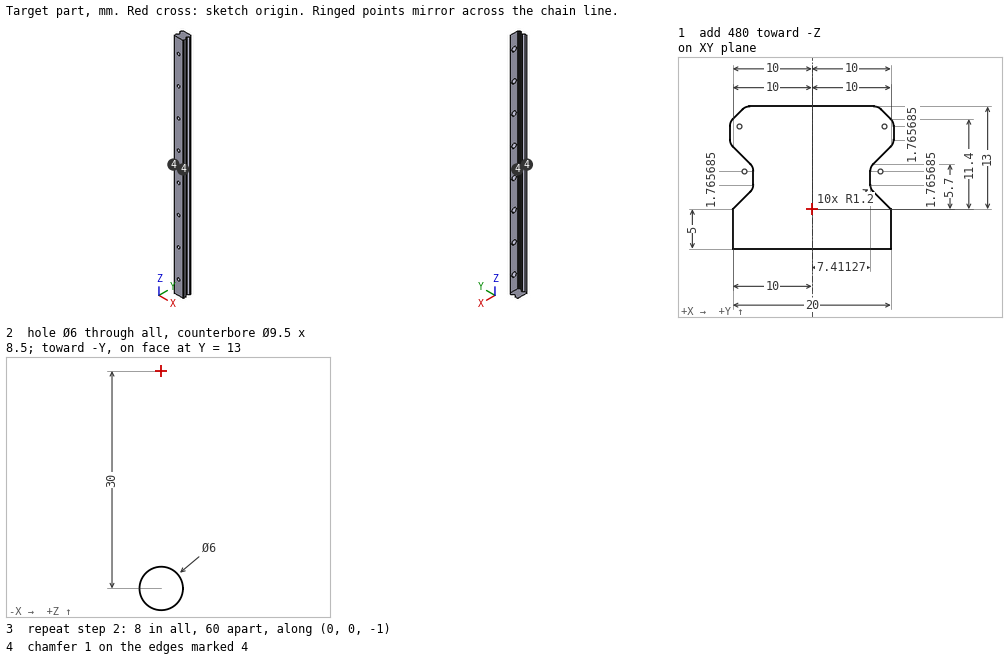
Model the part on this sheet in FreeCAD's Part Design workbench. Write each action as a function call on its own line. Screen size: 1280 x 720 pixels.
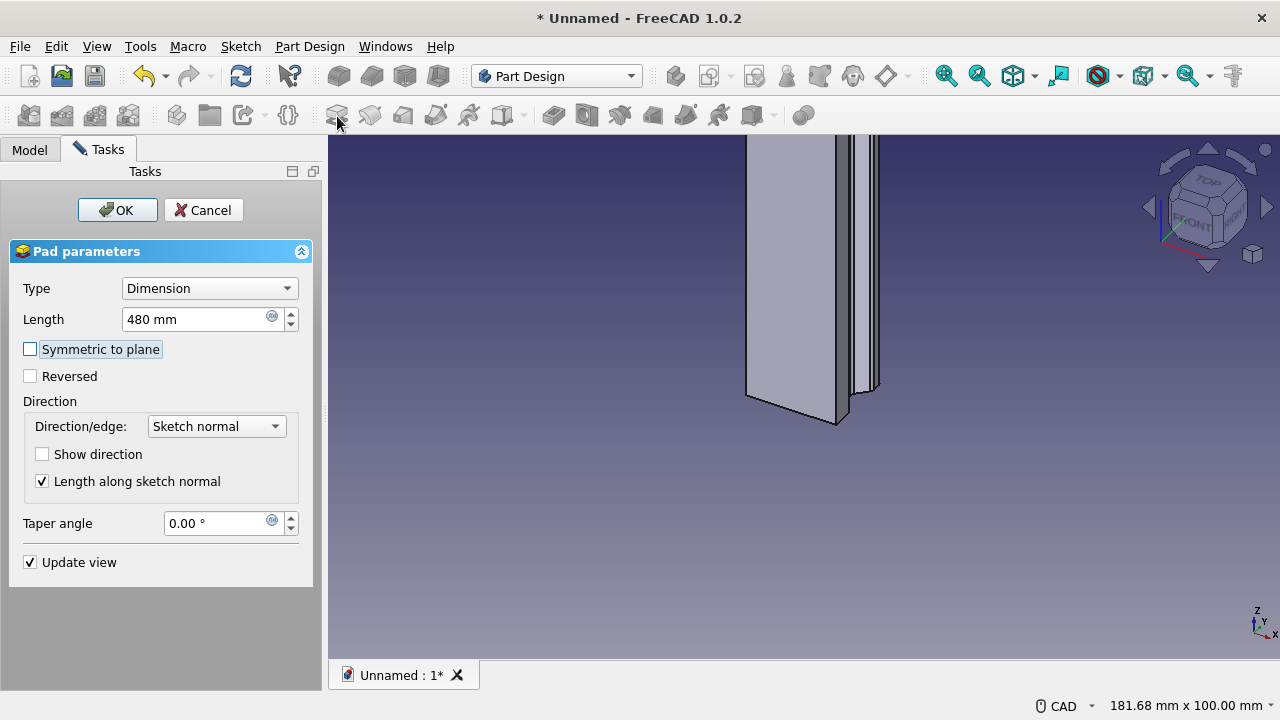
click(31, 376)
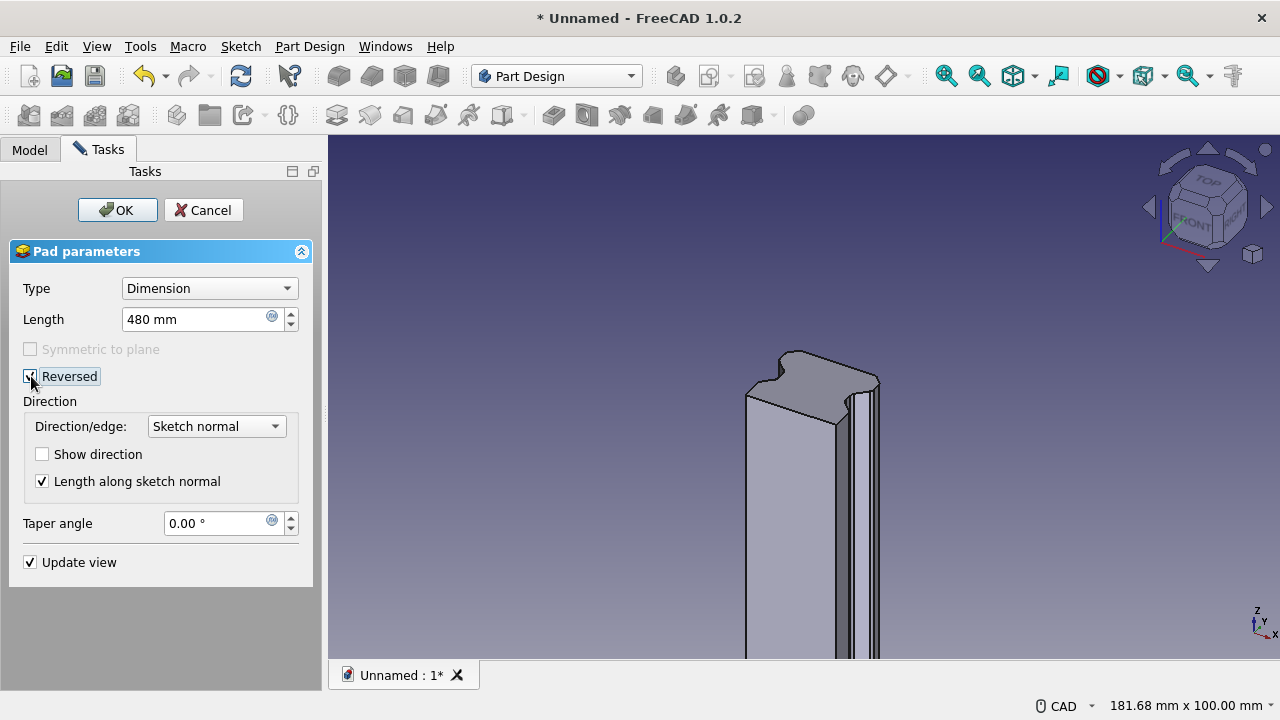
click(118, 210)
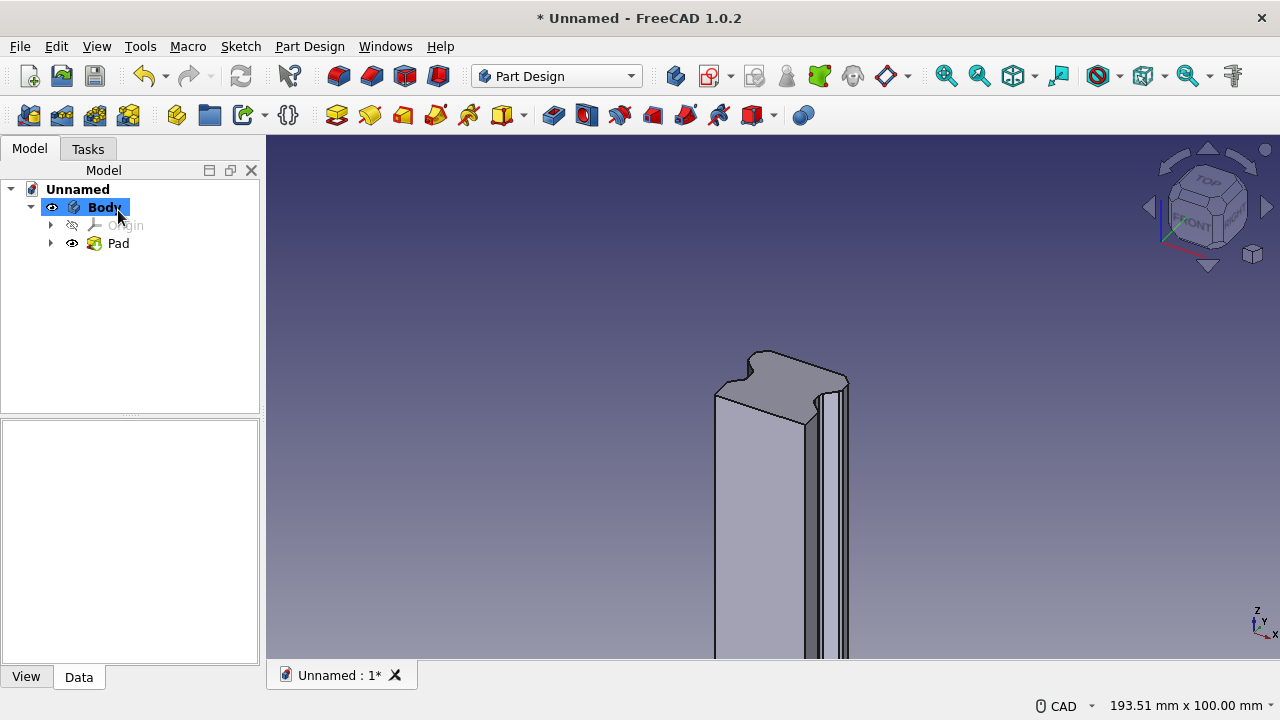
key(v)
key(f)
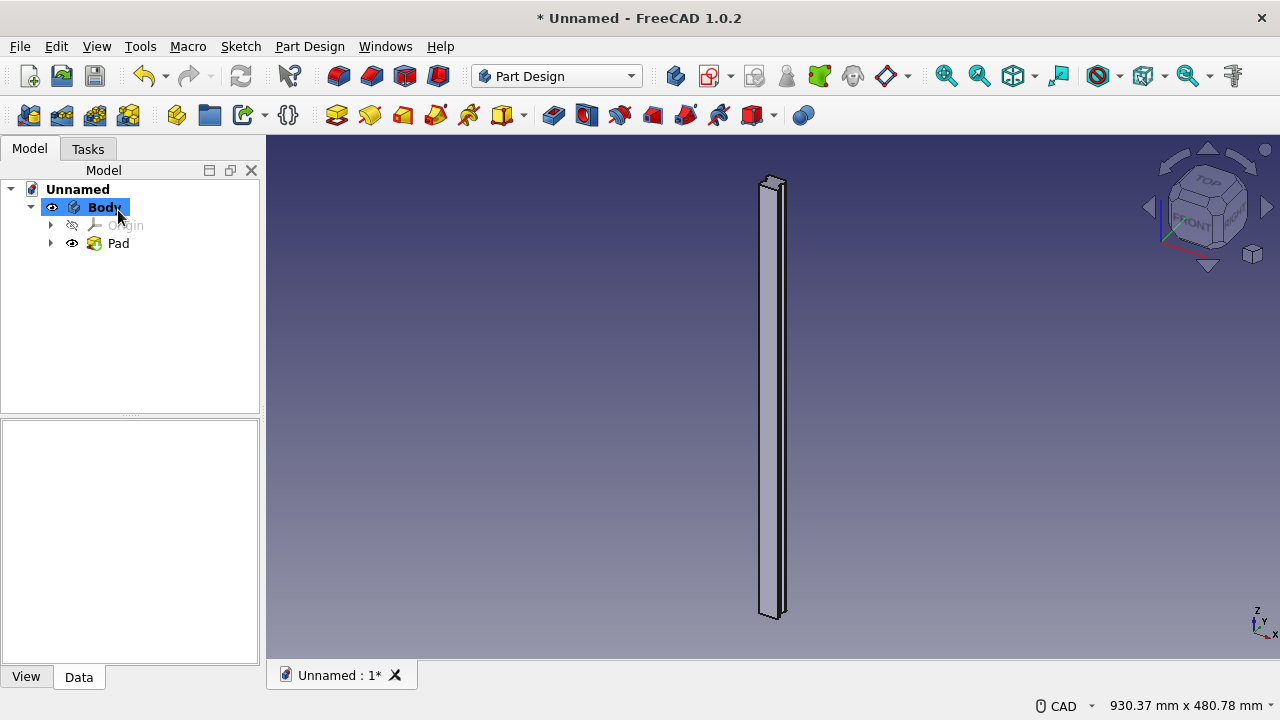
key(4)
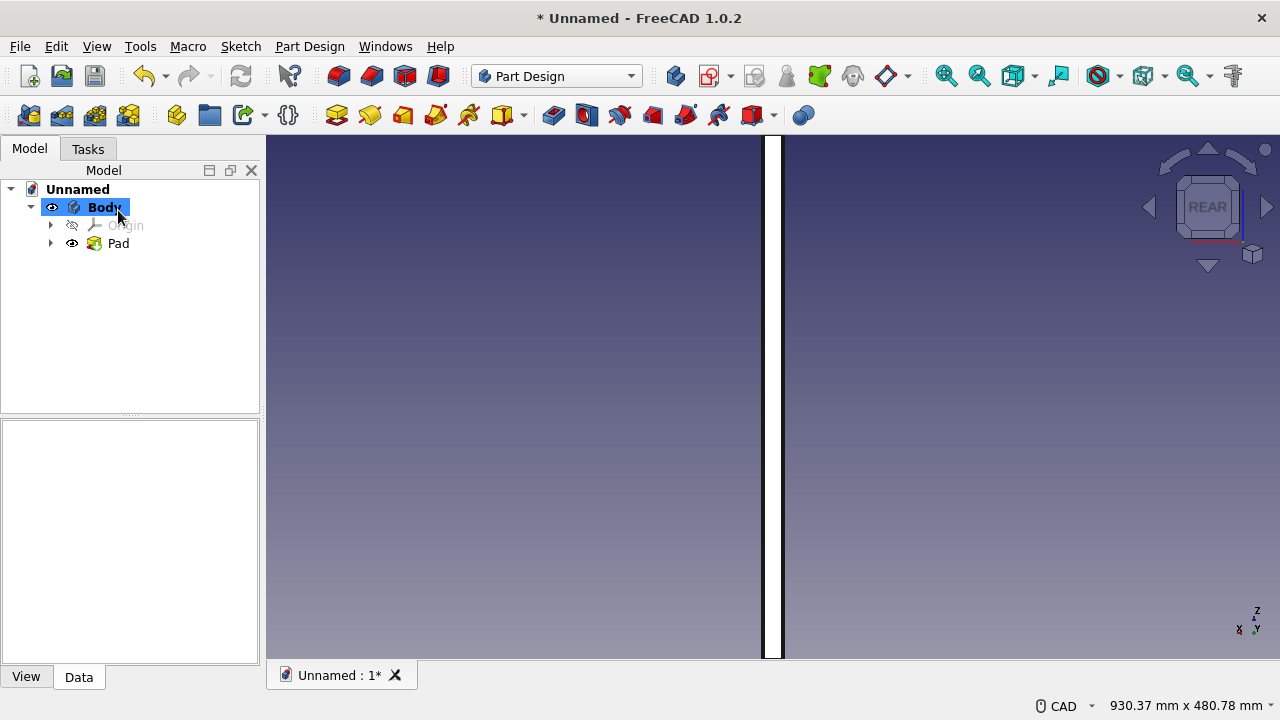
key(v)
key(f)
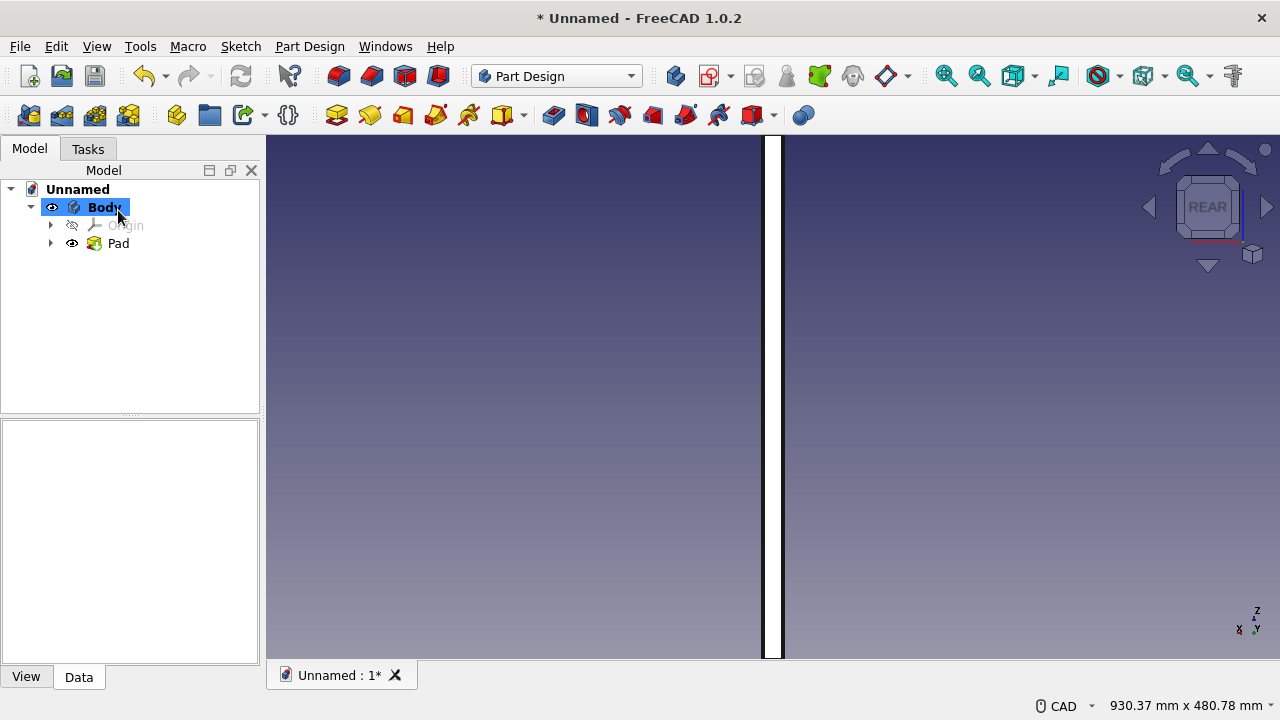
click(773, 172)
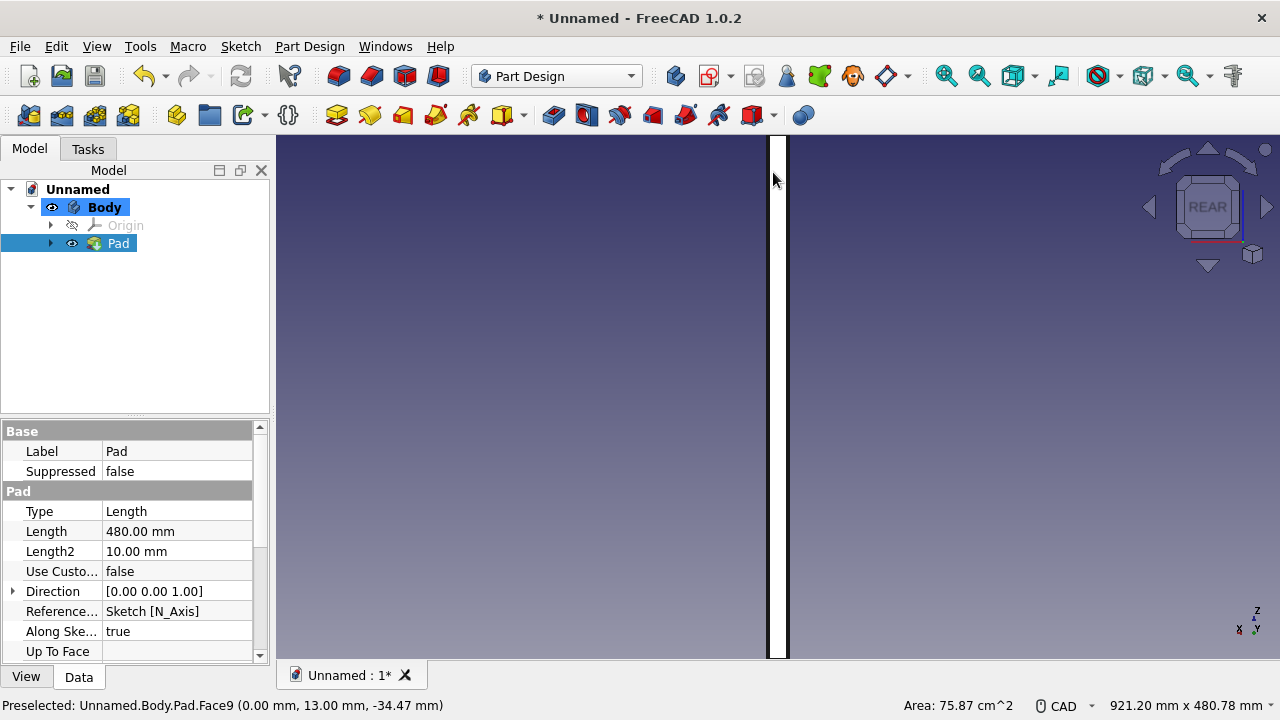
click(708, 76)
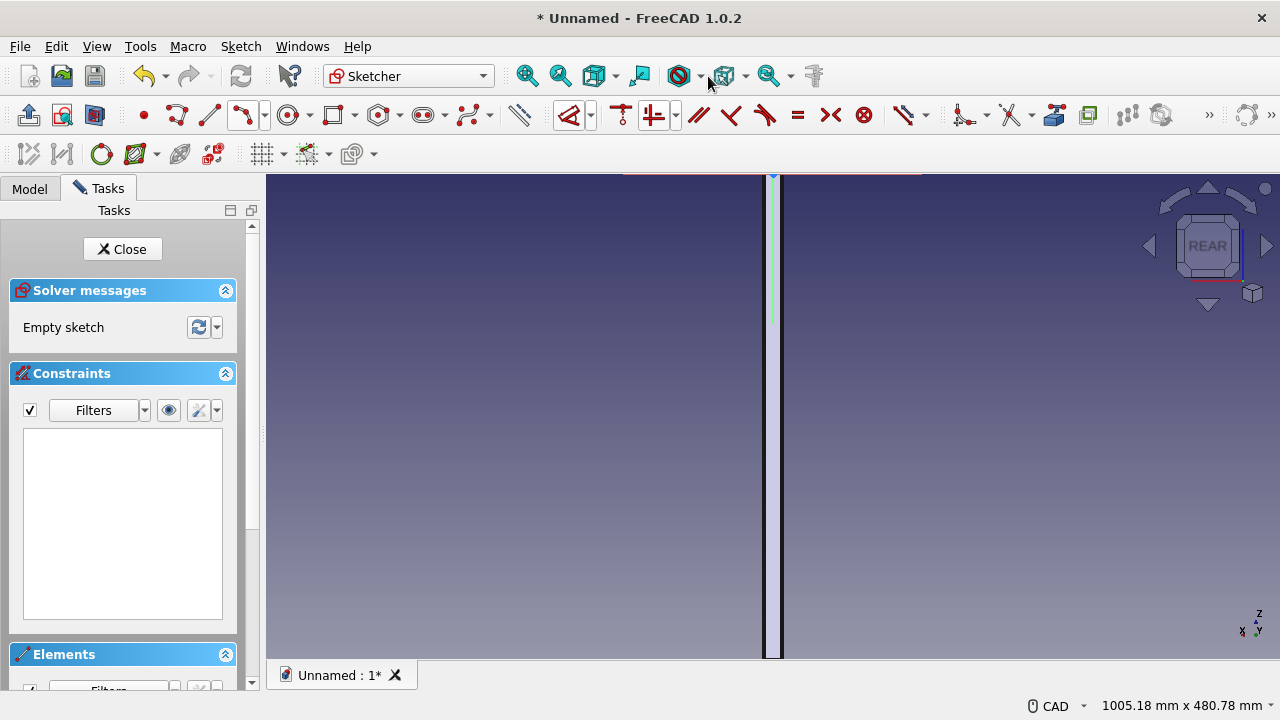
scroll(704, 416, down, 5)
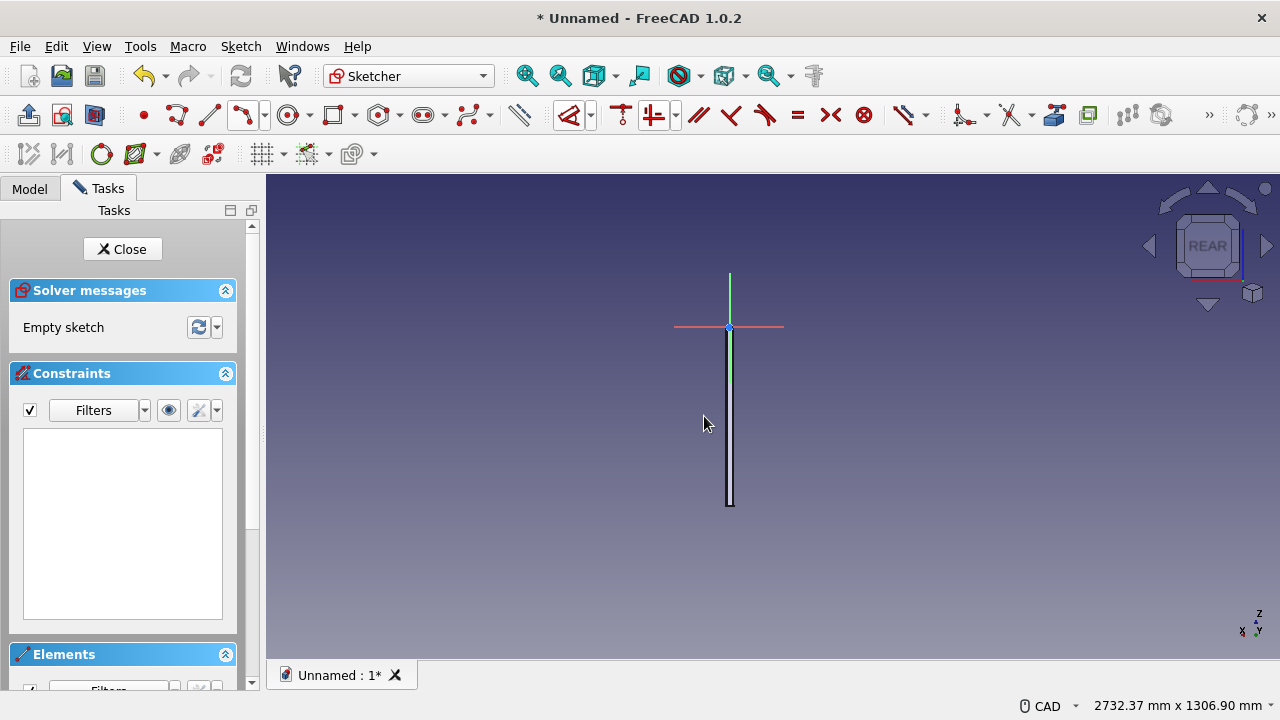
scroll(731, 334, up, 15)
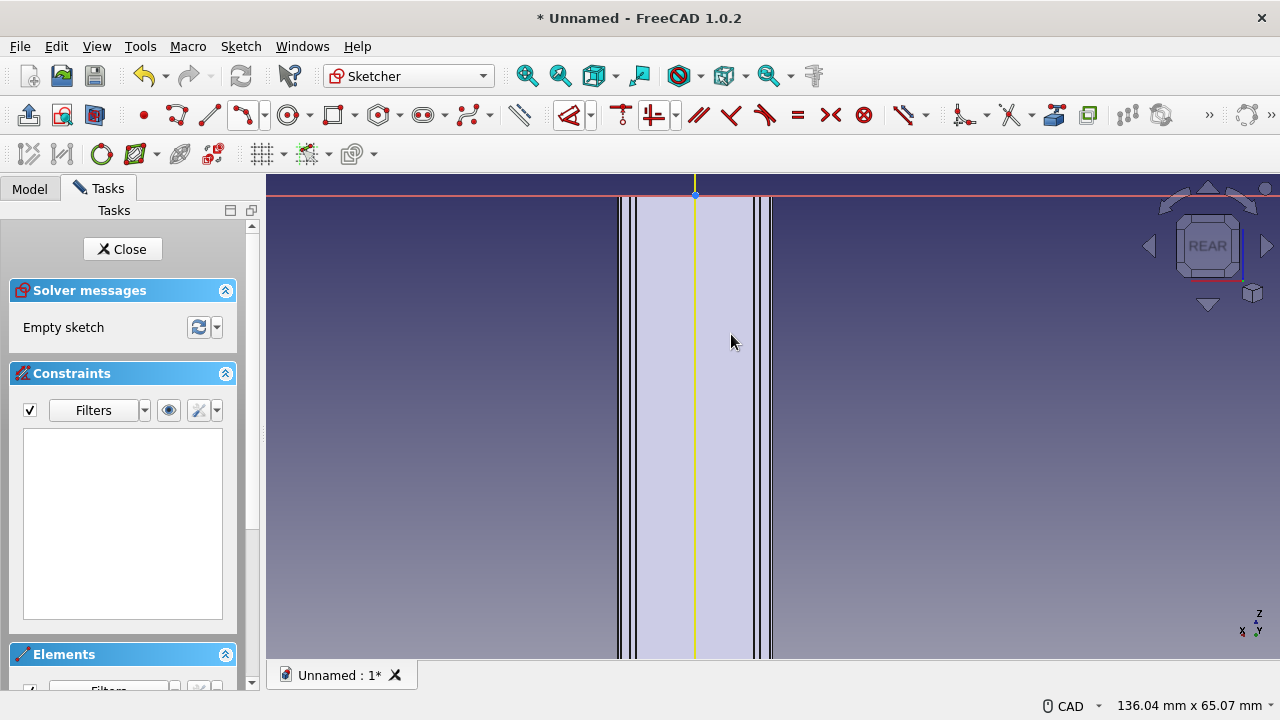
scroll(694, 420, up, 10)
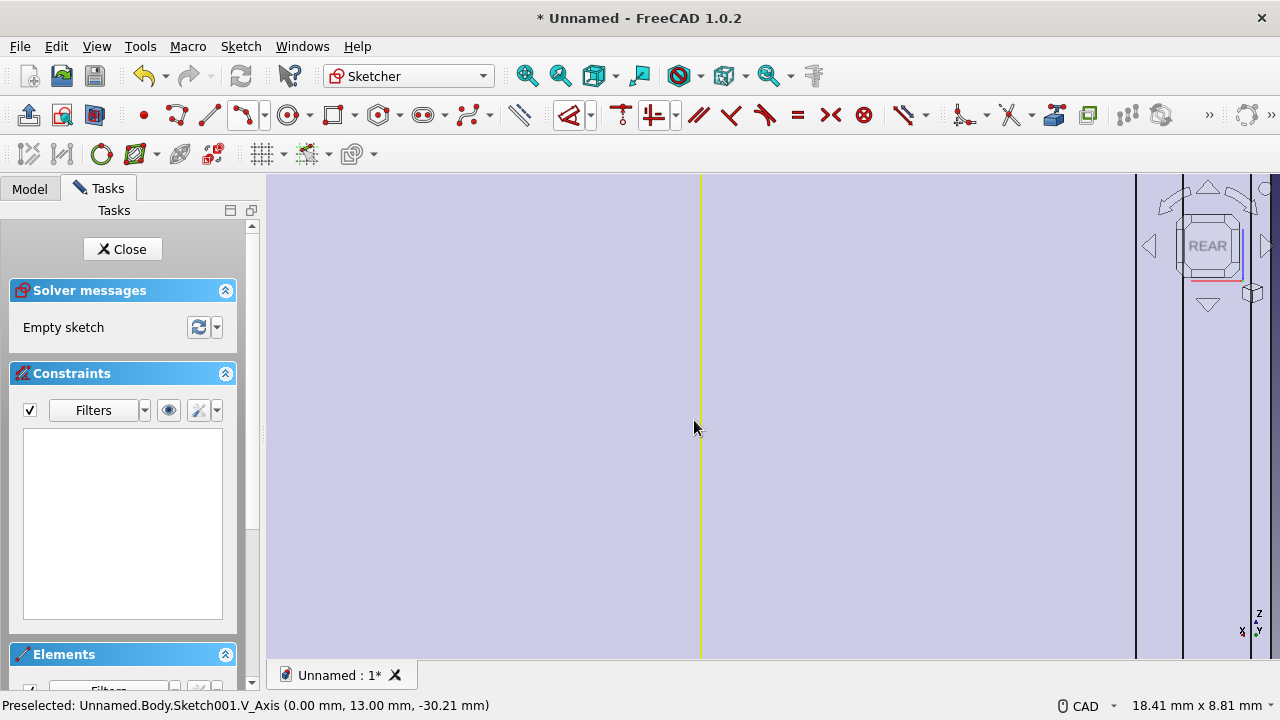
click(288, 116)